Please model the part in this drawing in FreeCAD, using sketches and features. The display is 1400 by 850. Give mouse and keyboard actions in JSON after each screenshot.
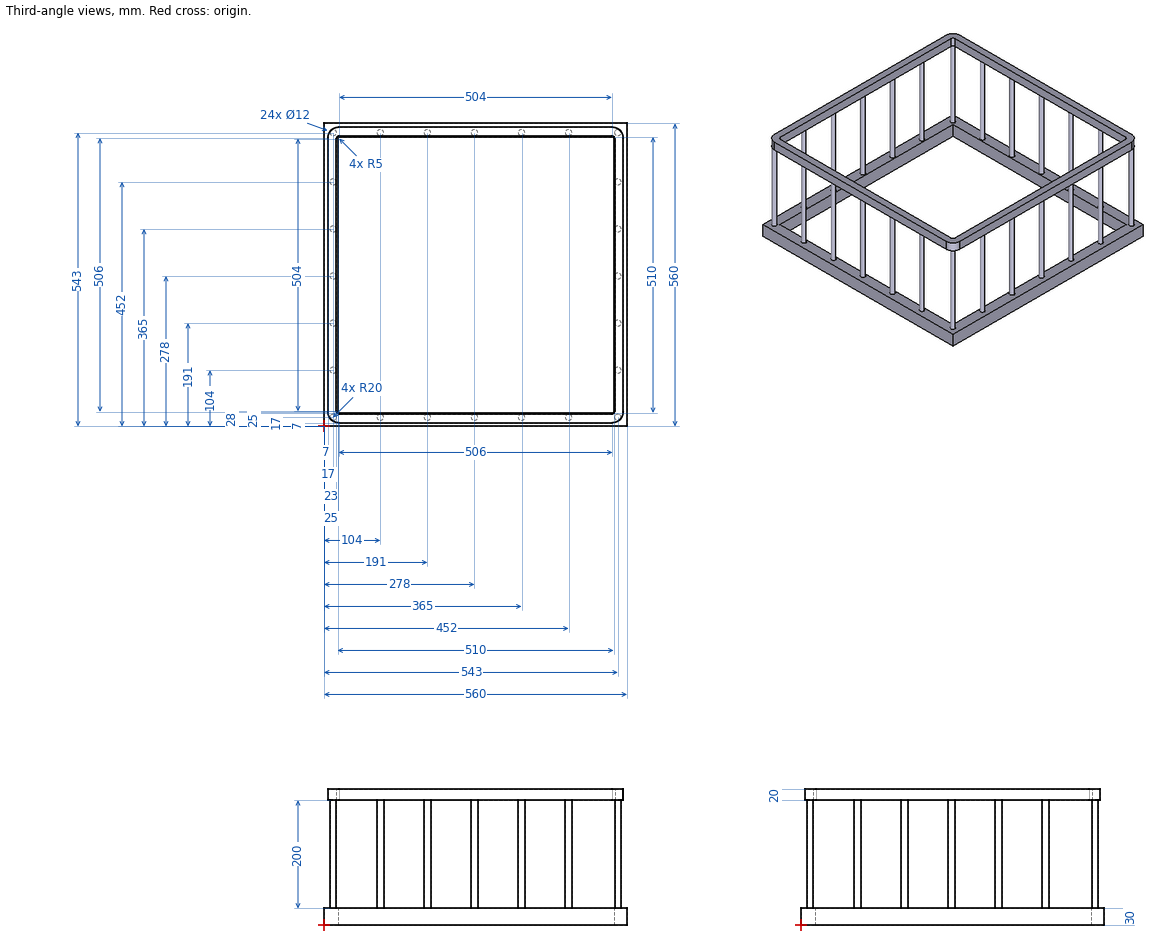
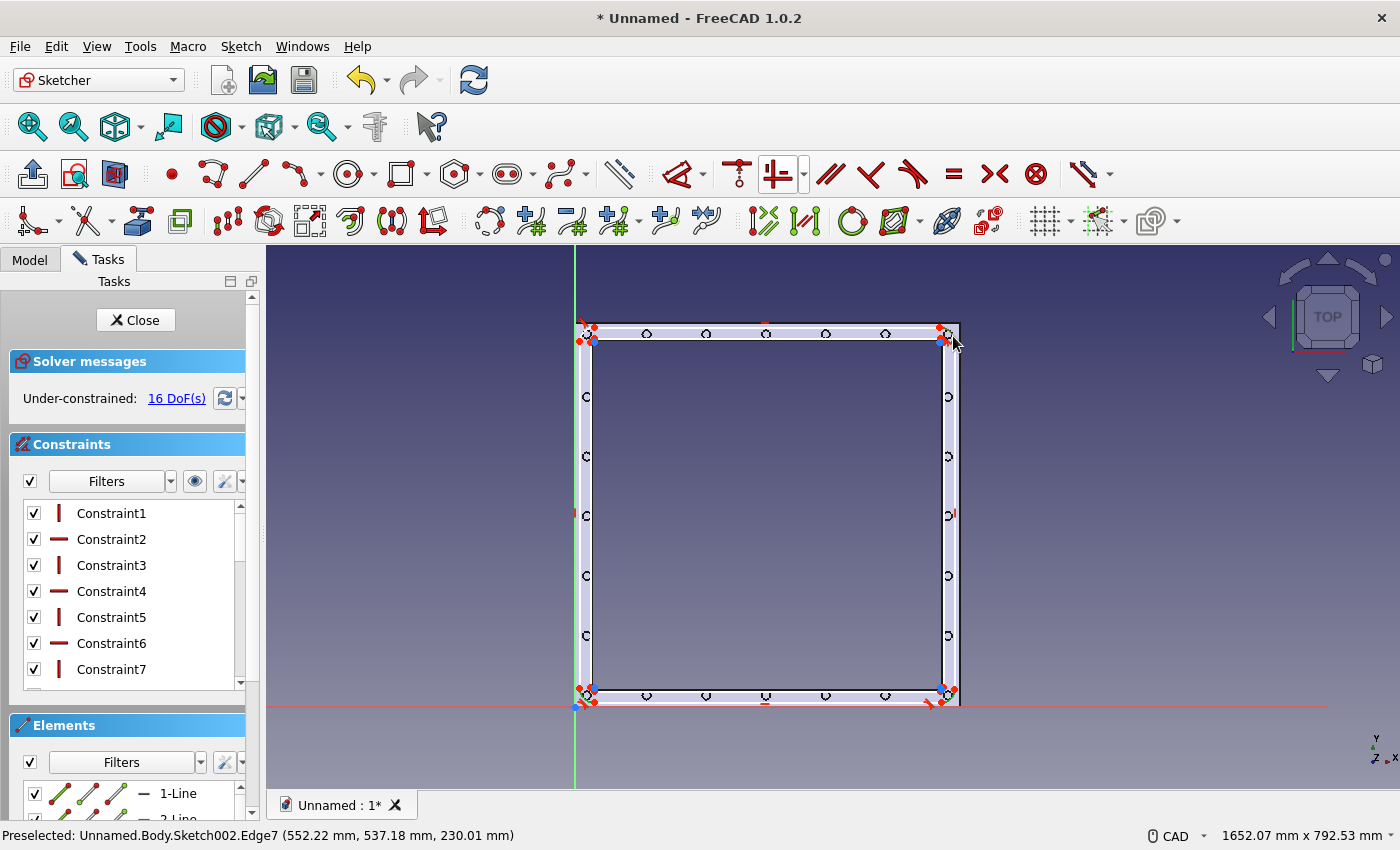
{"action": "scroll", "coordinate": [588, 329], "scroll_direction": "up", "scroll_amount": 4}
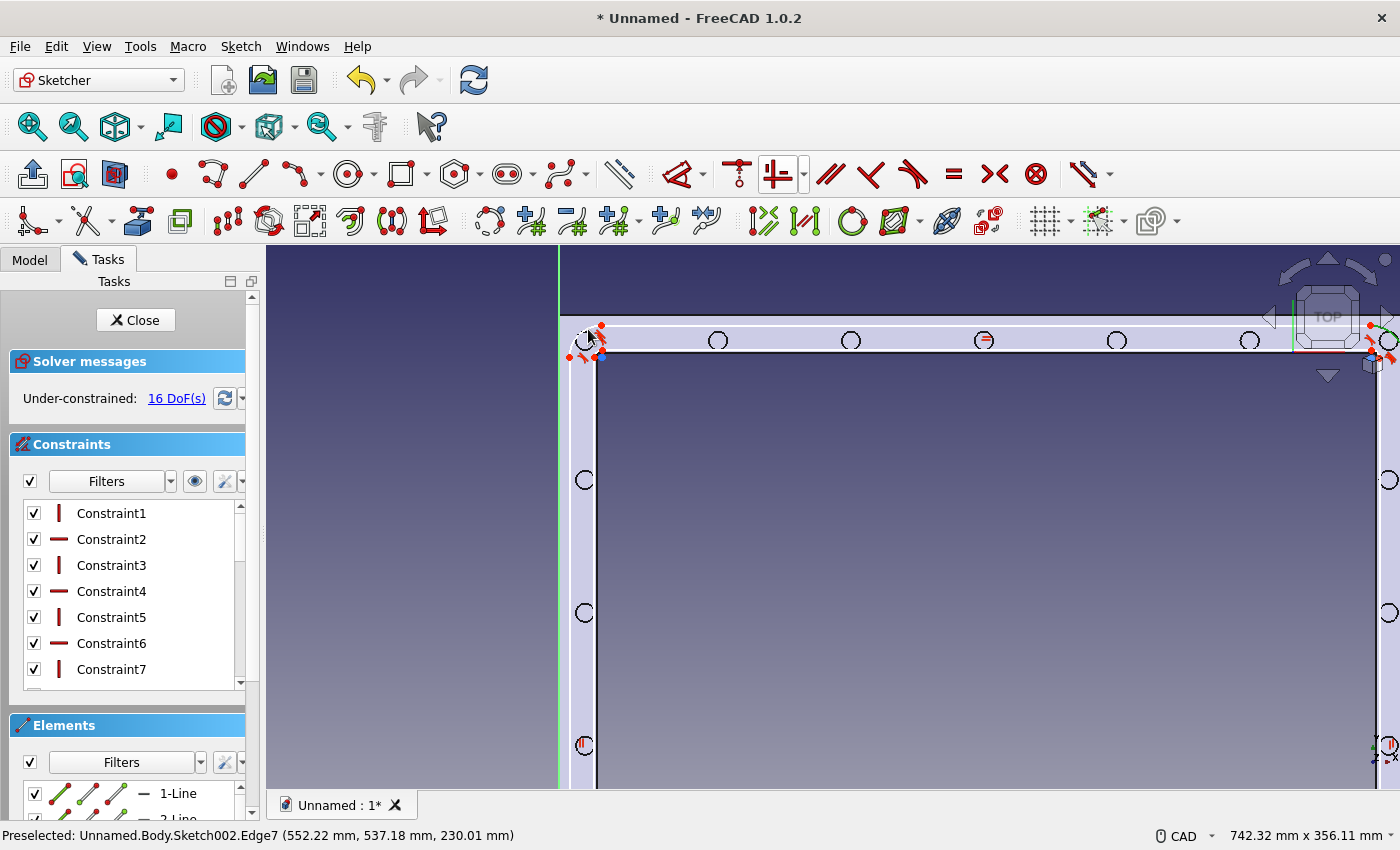
{"action": "left_click", "coordinate": [587, 329]}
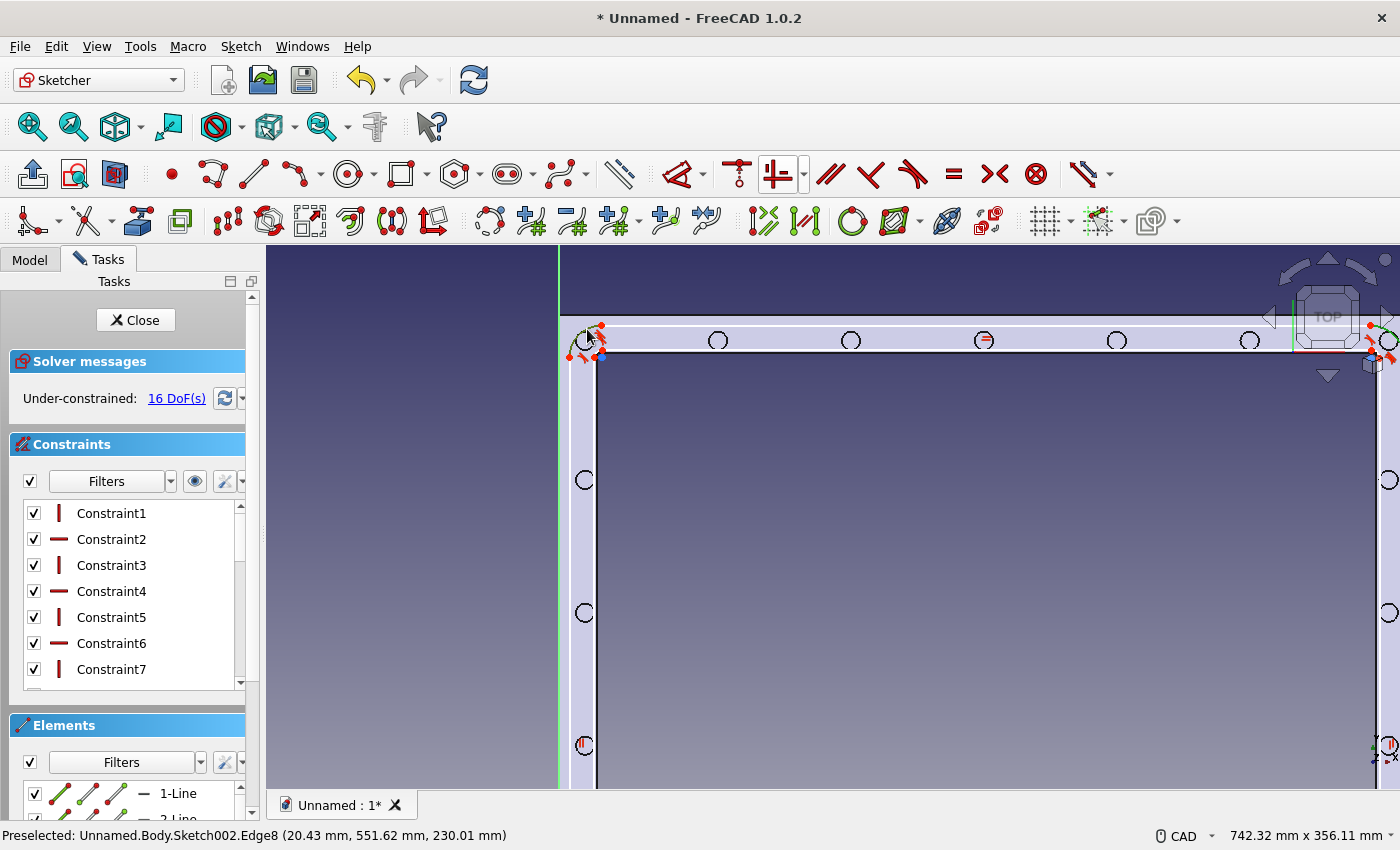
{"action": "left_click", "coordinate": [954, 174]}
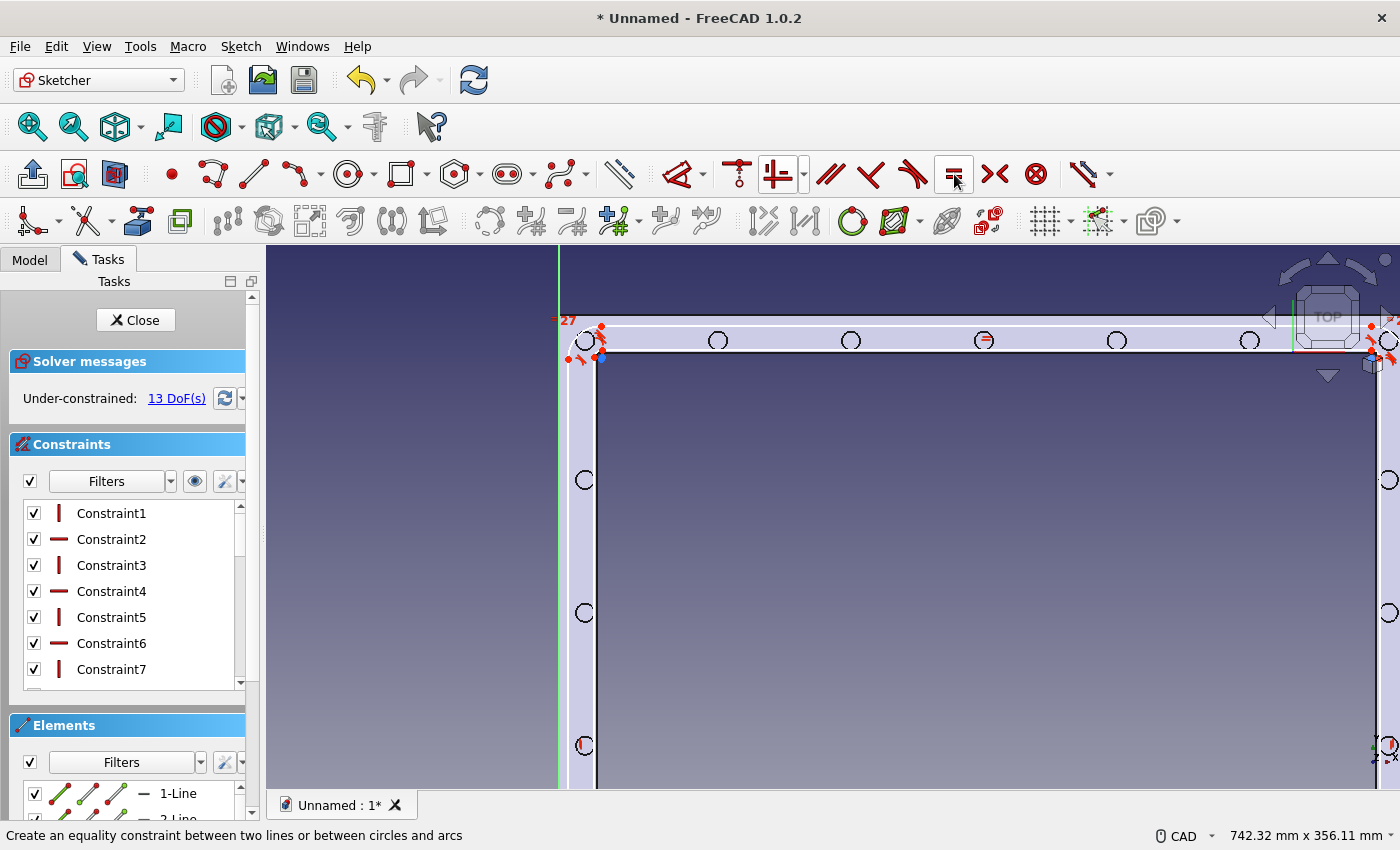
{"action": "scroll", "coordinate": [597, 352], "scroll_direction": "up", "scroll_amount": 5}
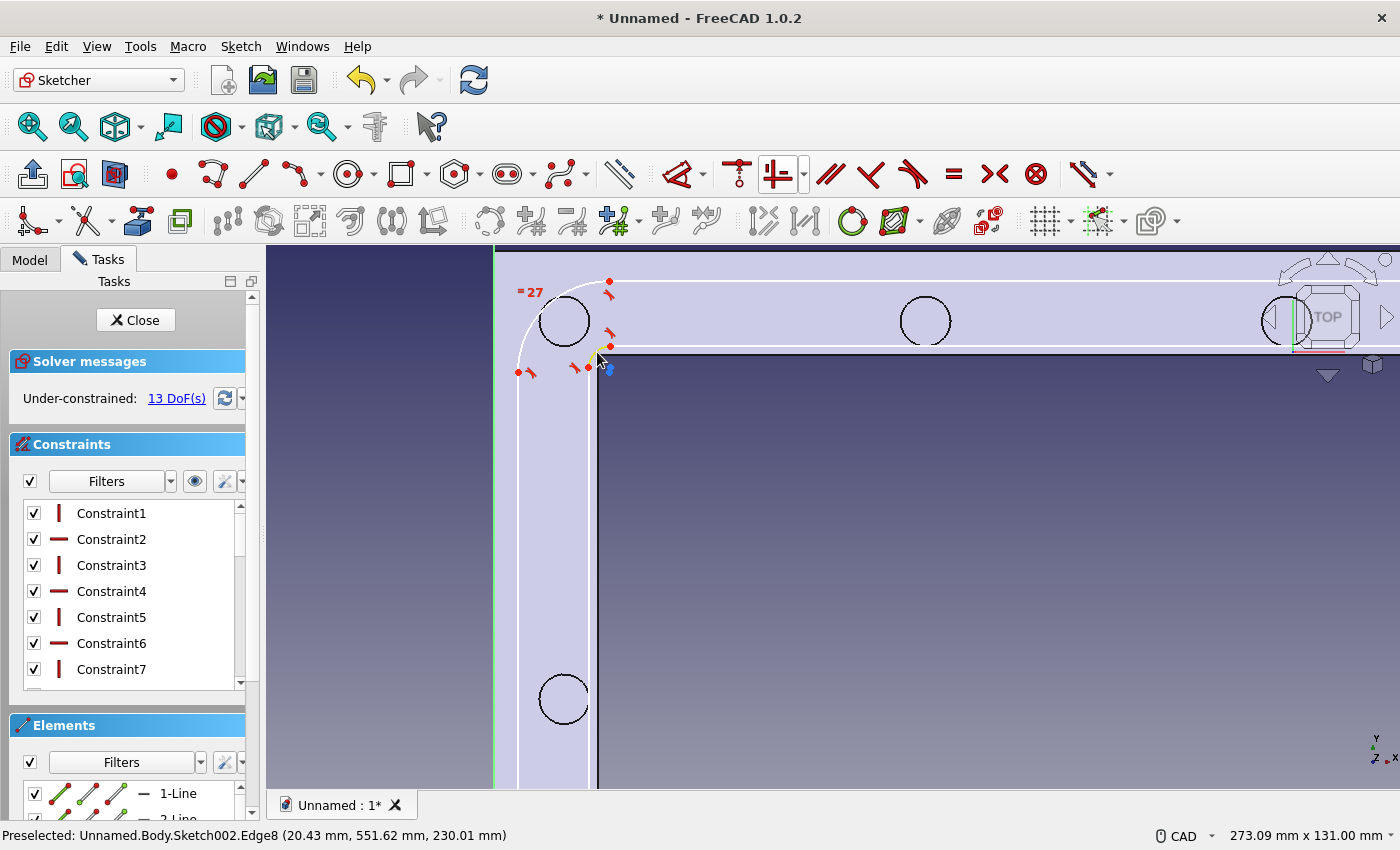
{"action": "left_click", "coordinate": [595, 353]}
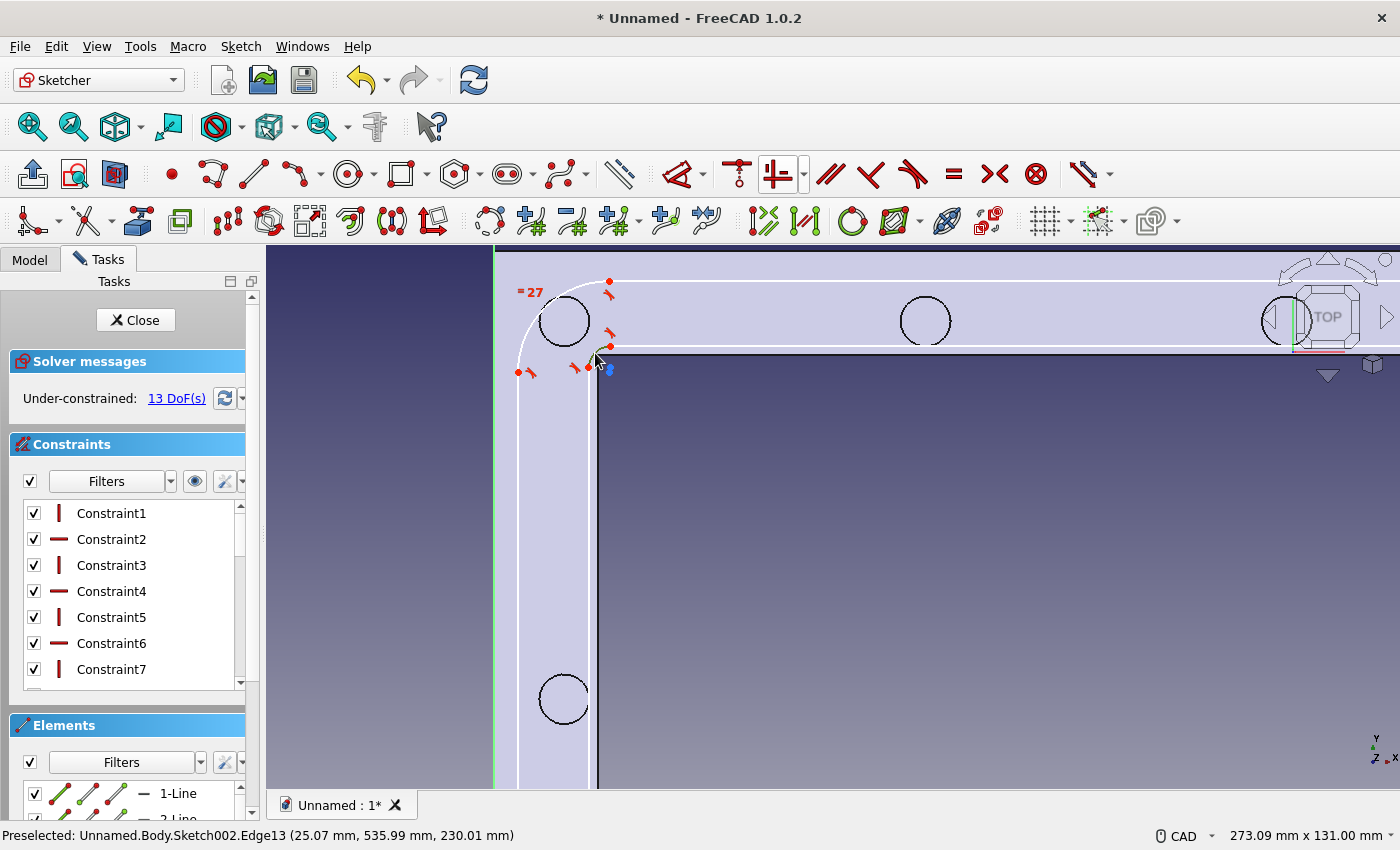
{"action": "scroll", "coordinate": [591, 337], "scroll_direction": "down", "scroll_amount": 9}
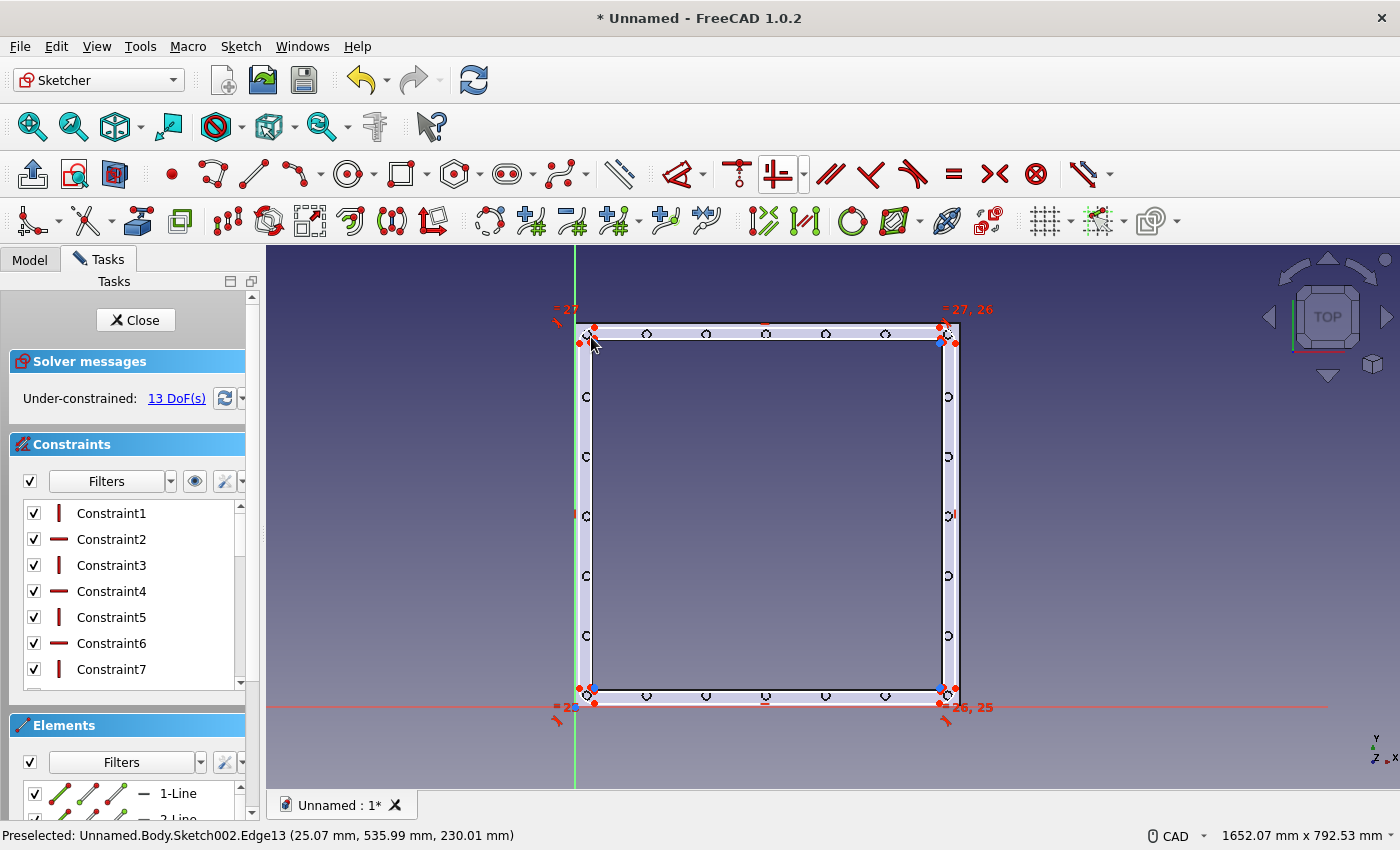
{"action": "scroll", "coordinate": [944, 341], "scroll_direction": "up", "scroll_amount": 11}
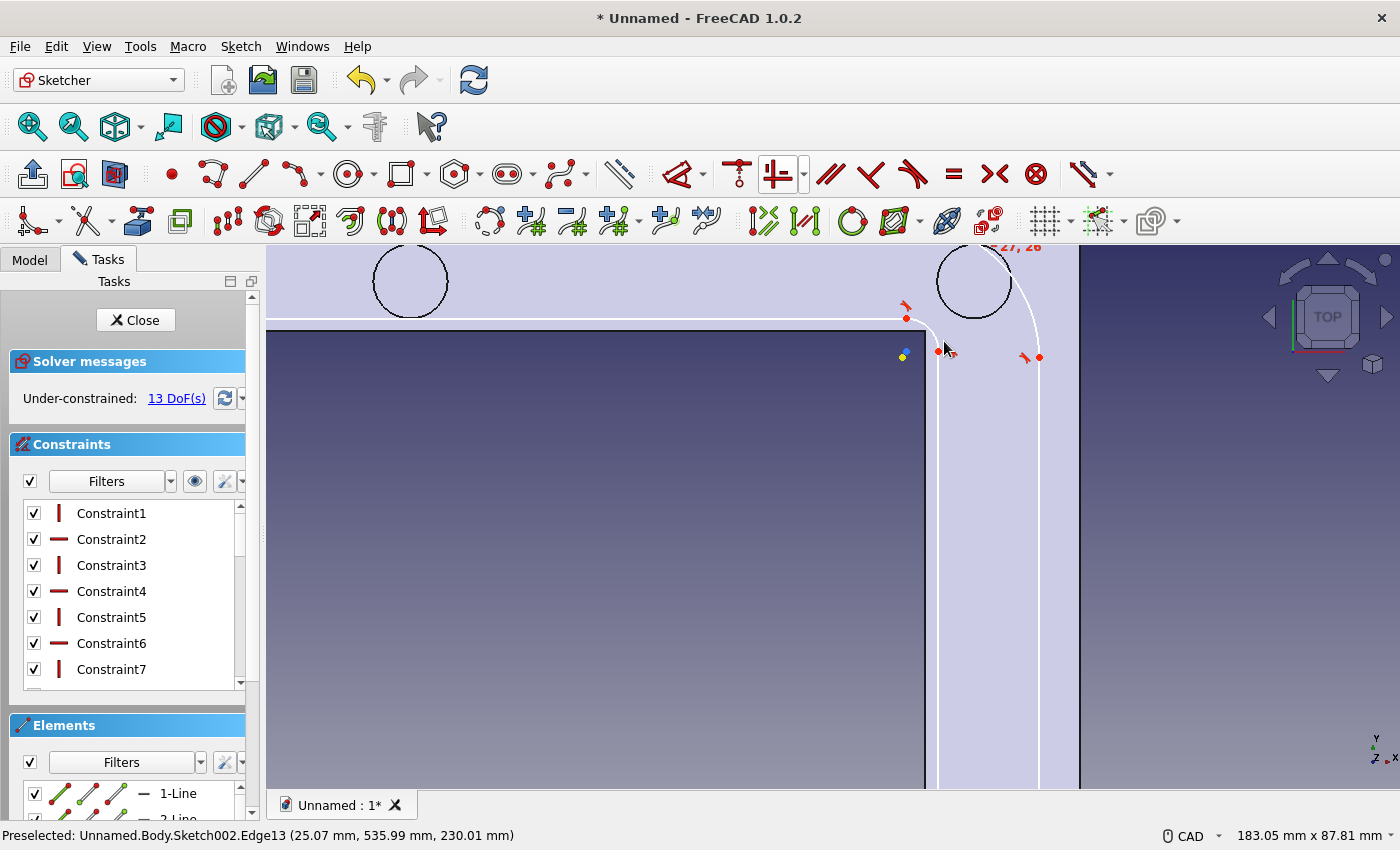
{"action": "left_click", "coordinate": [935, 336]}